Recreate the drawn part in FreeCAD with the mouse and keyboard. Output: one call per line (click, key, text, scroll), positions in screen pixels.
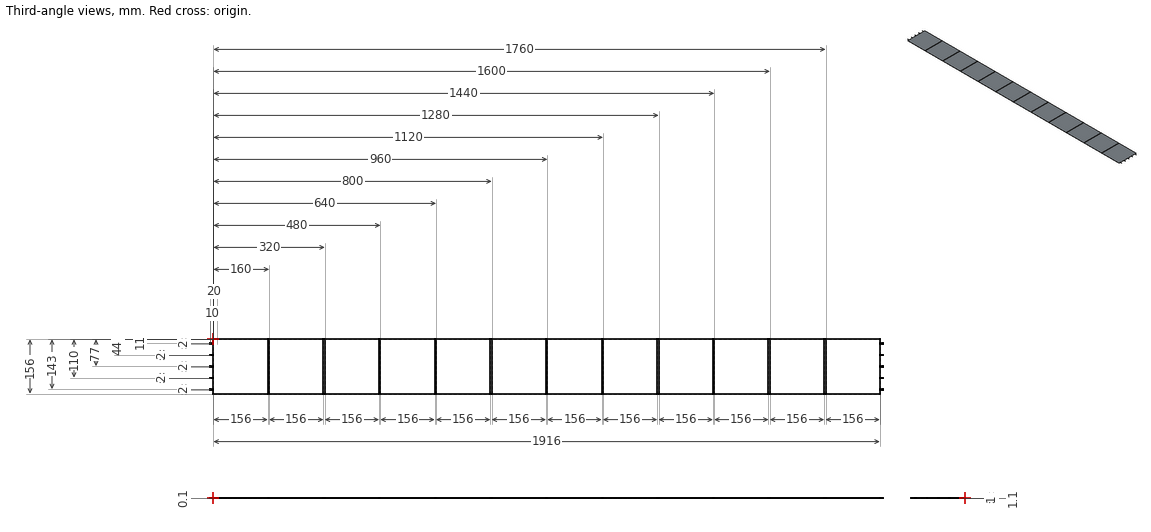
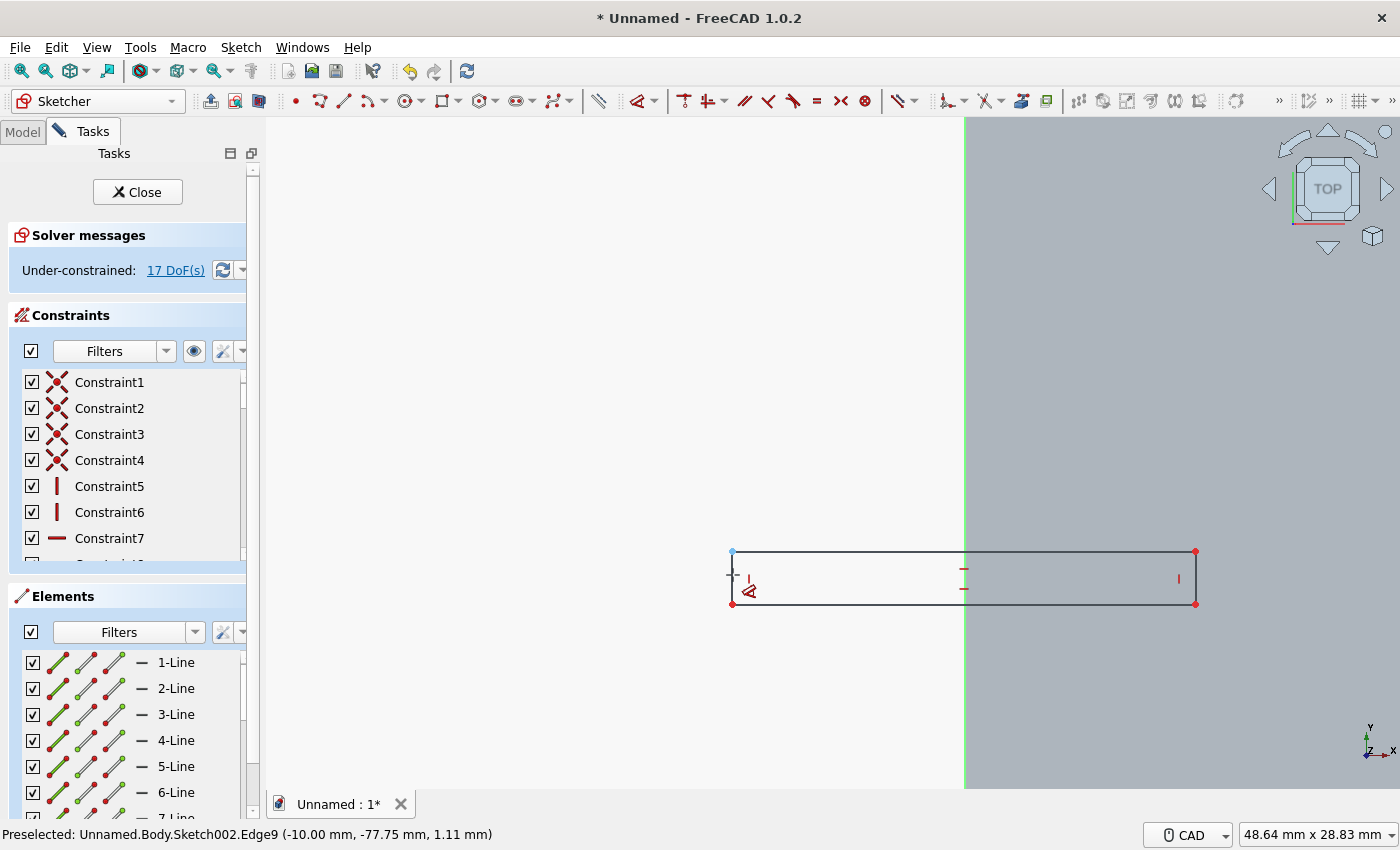
click(732, 568)
click(698, 578)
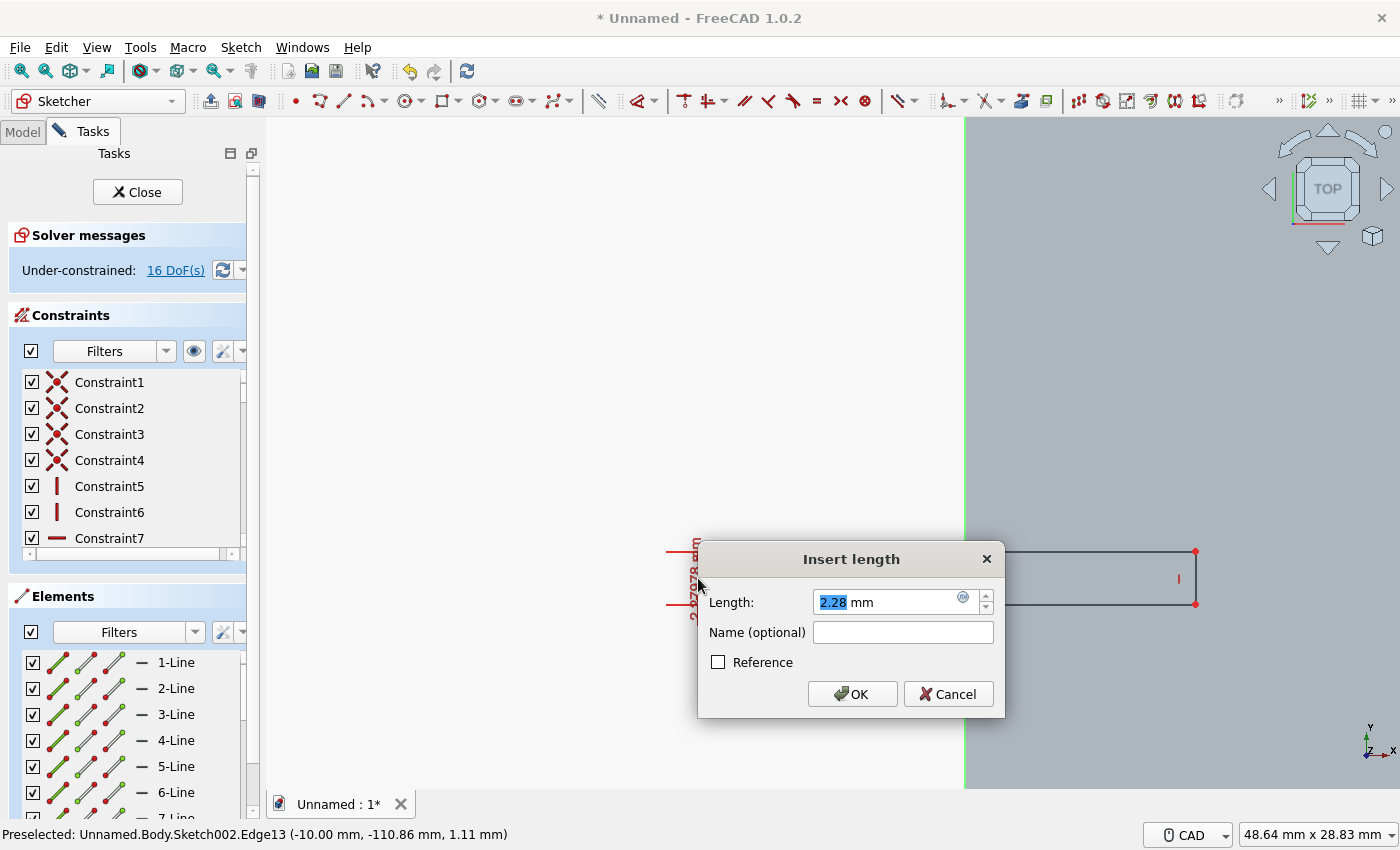
text(2)
key(Return)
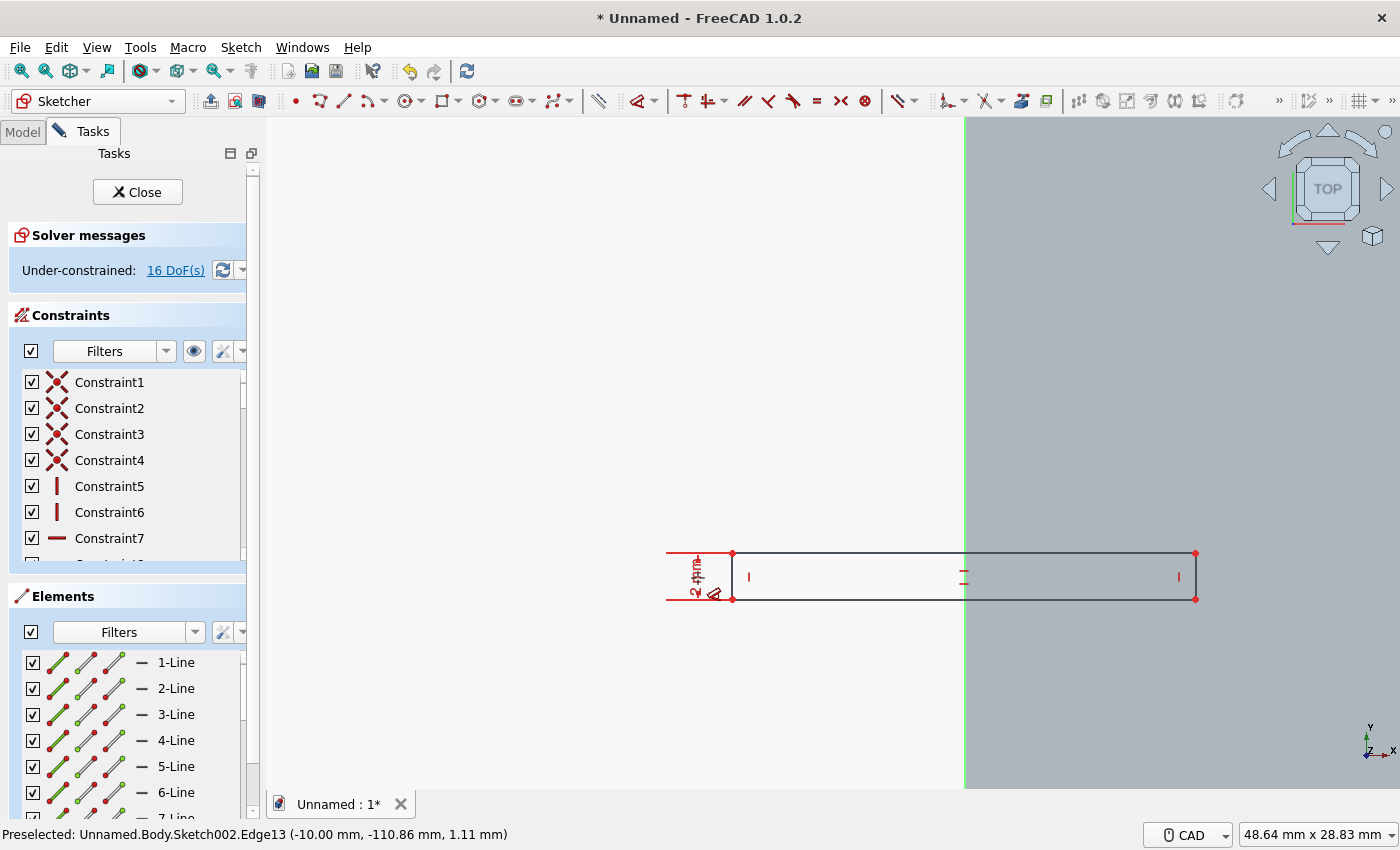
scroll(733, 575, down, 10)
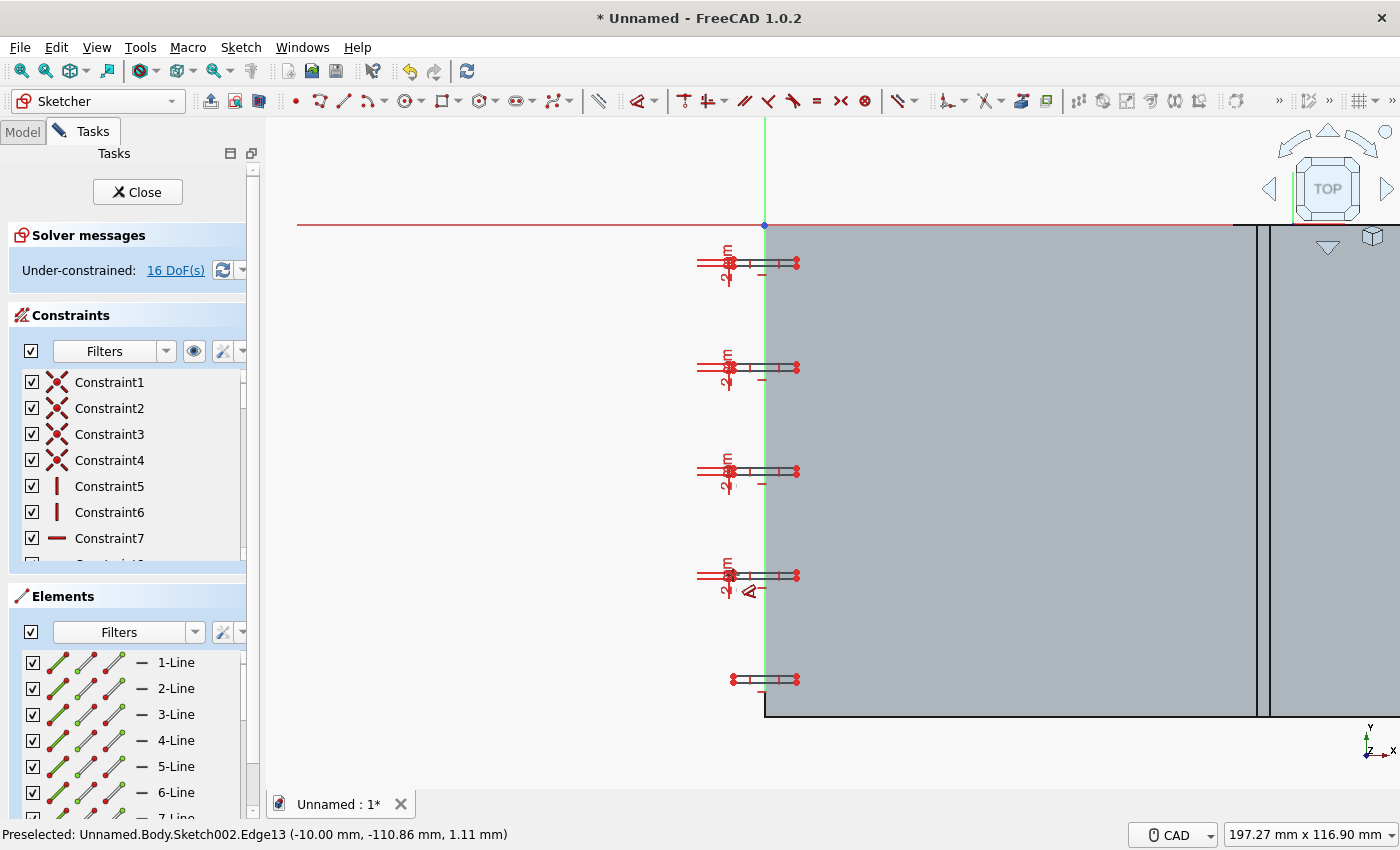
scroll(733, 678, up, 10)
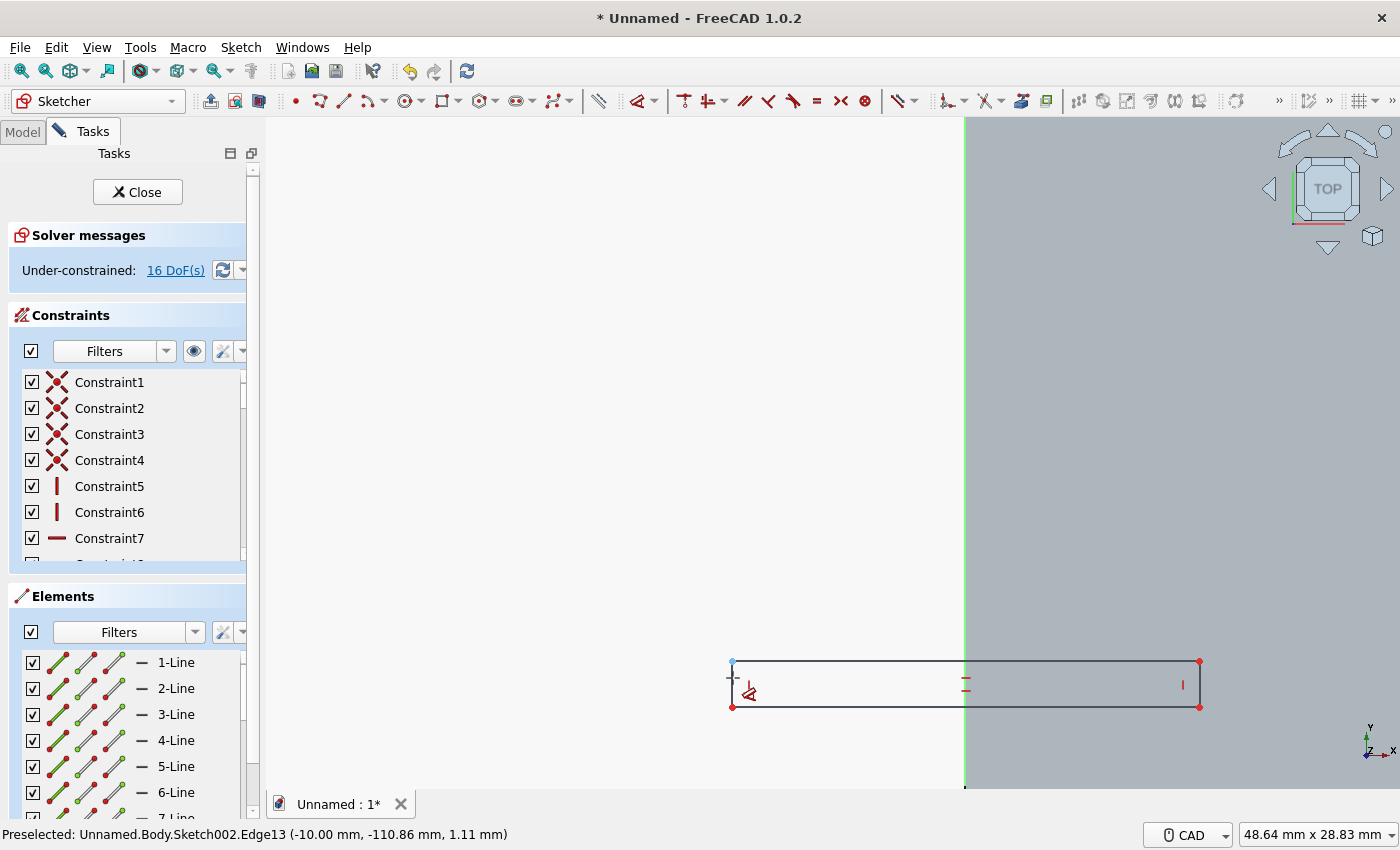
click(732, 675)
click(698, 684)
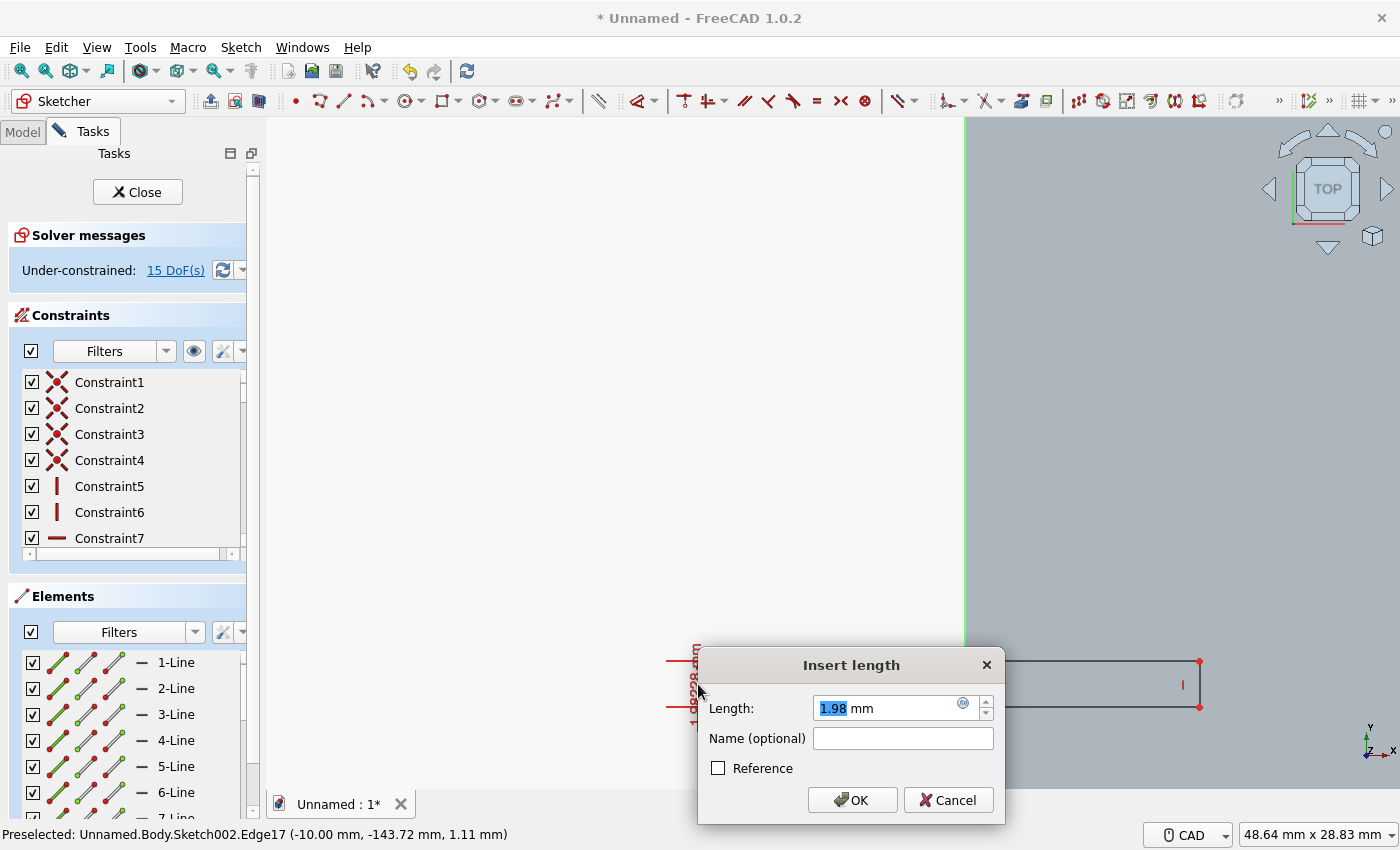
text(2)
key(Return)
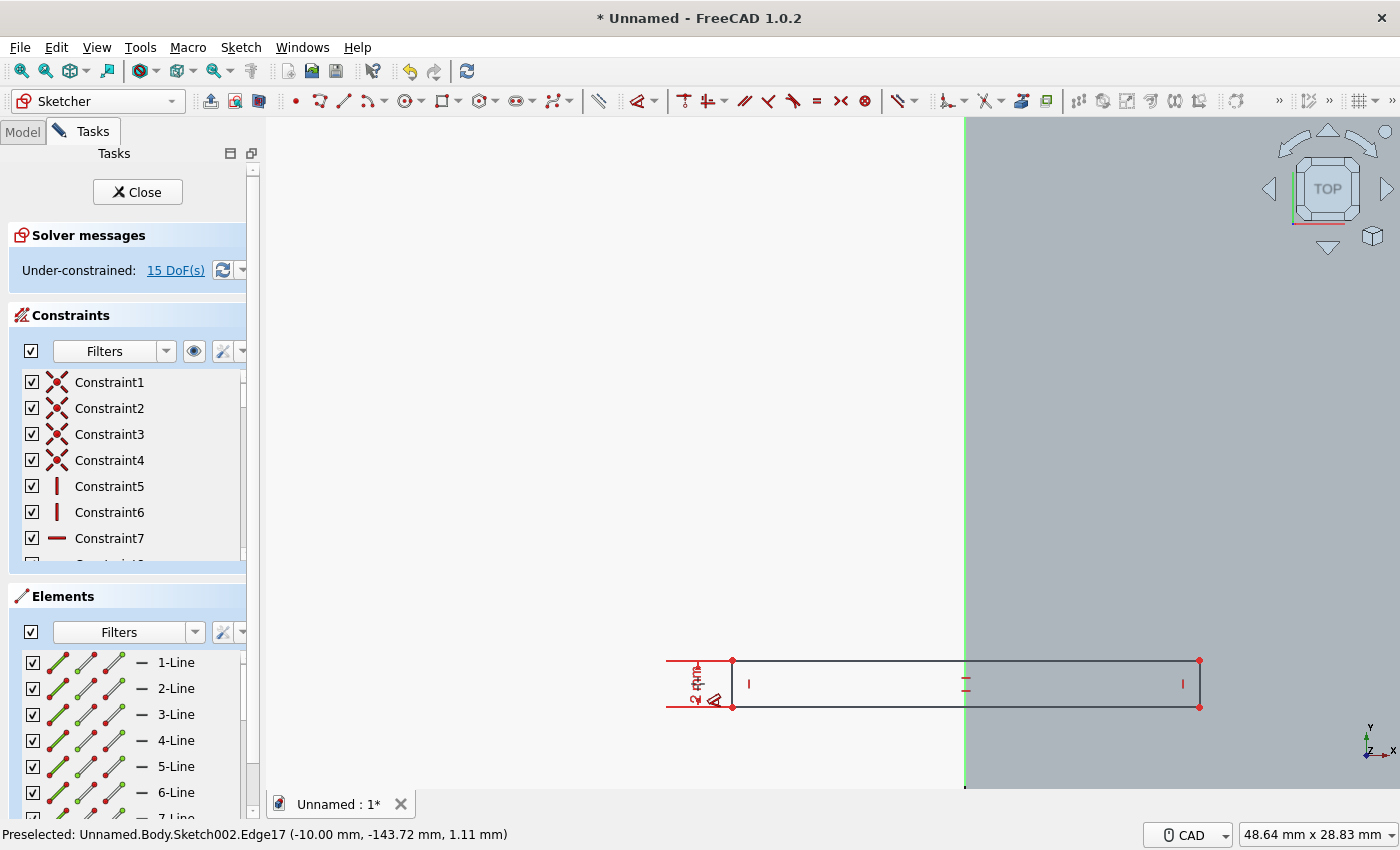
scroll(733, 678, down, 10)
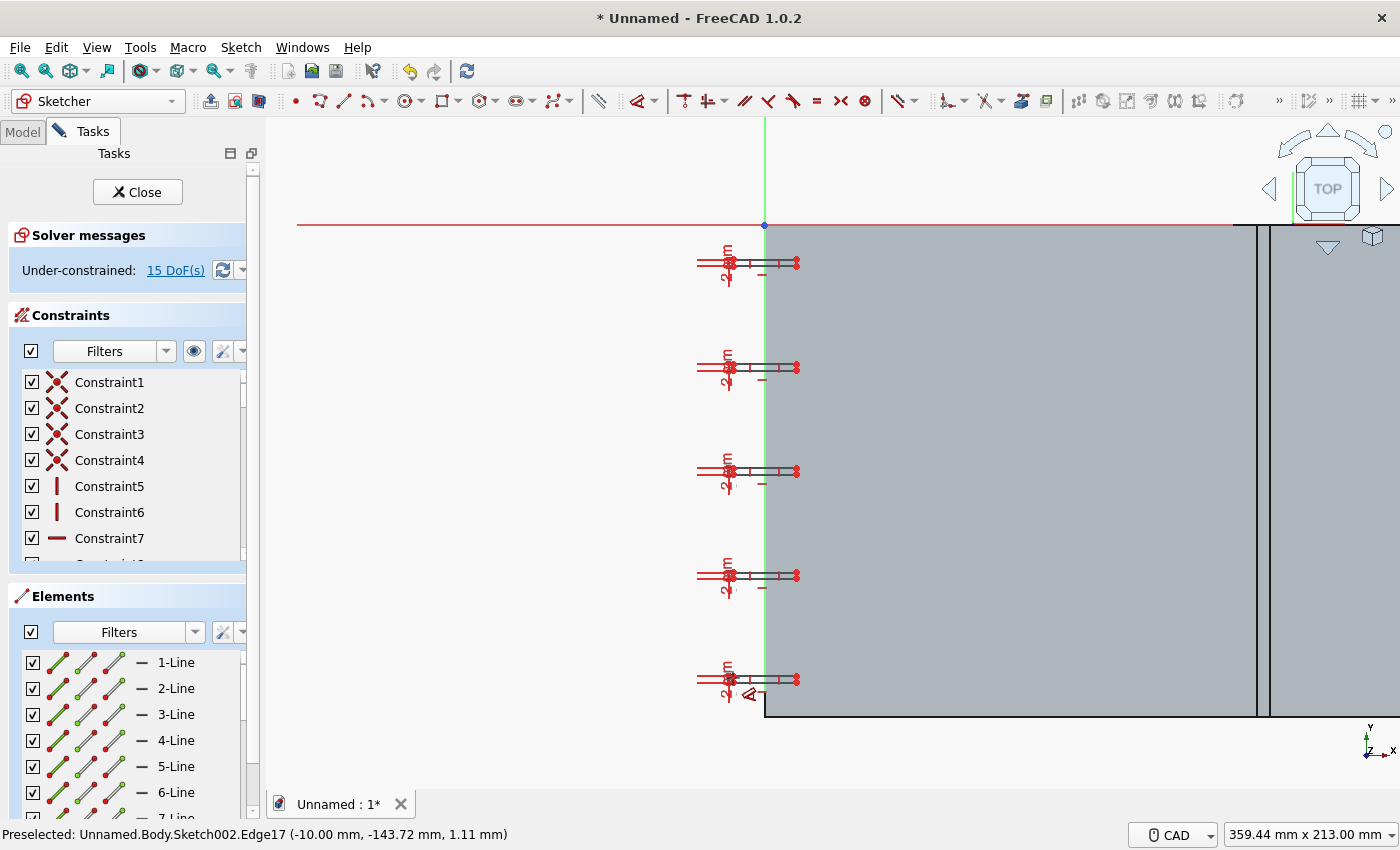
scroll(752, 266, up, 4)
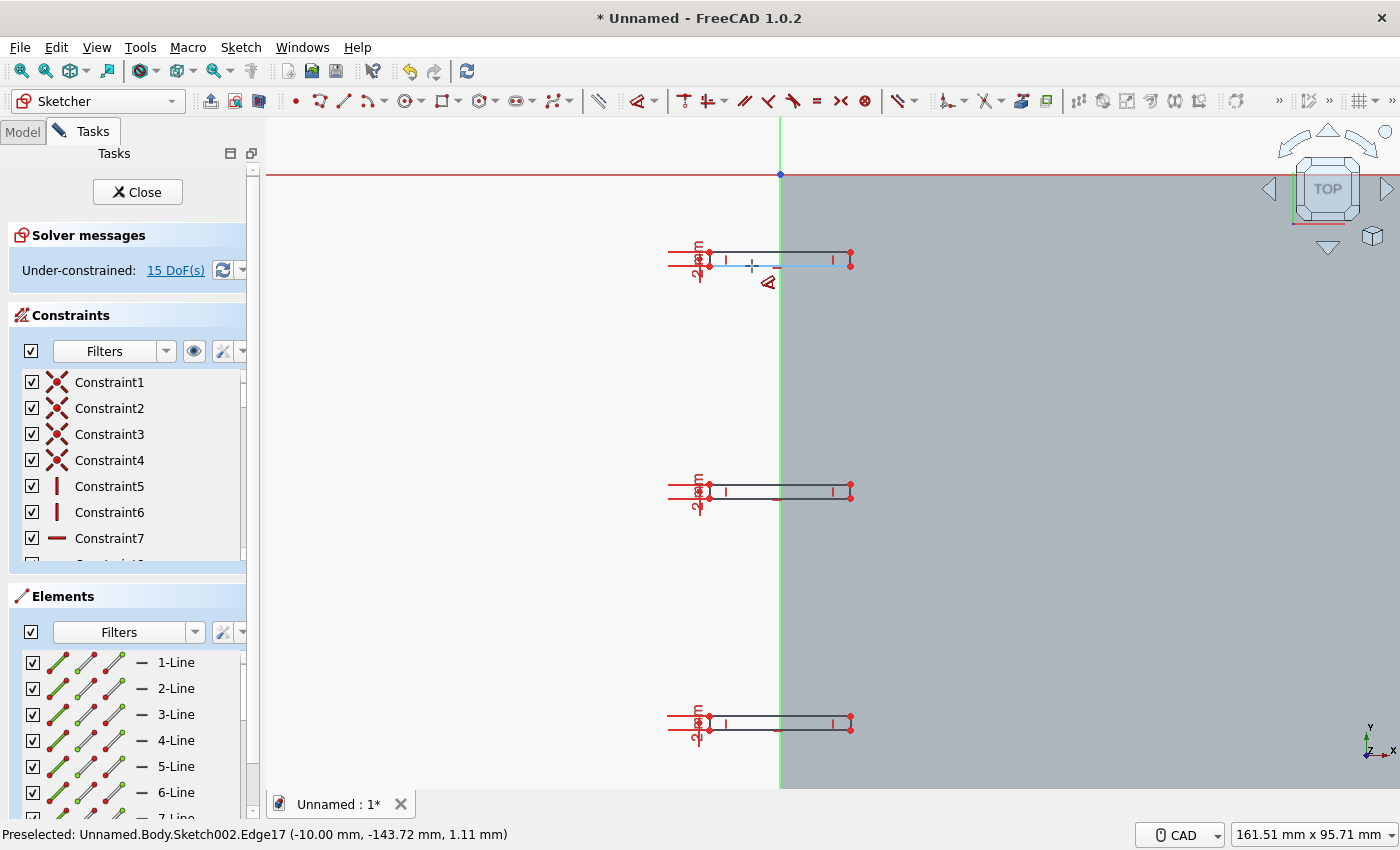
click(752, 266)
click(748, 232)